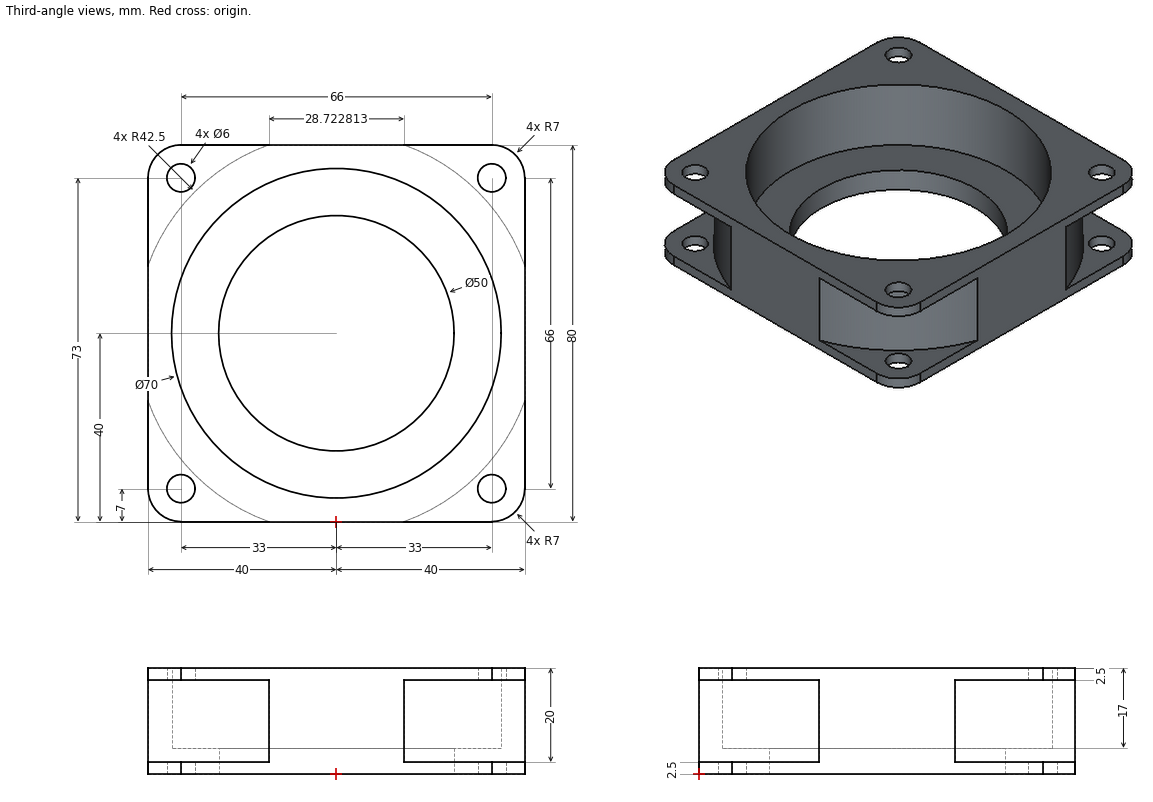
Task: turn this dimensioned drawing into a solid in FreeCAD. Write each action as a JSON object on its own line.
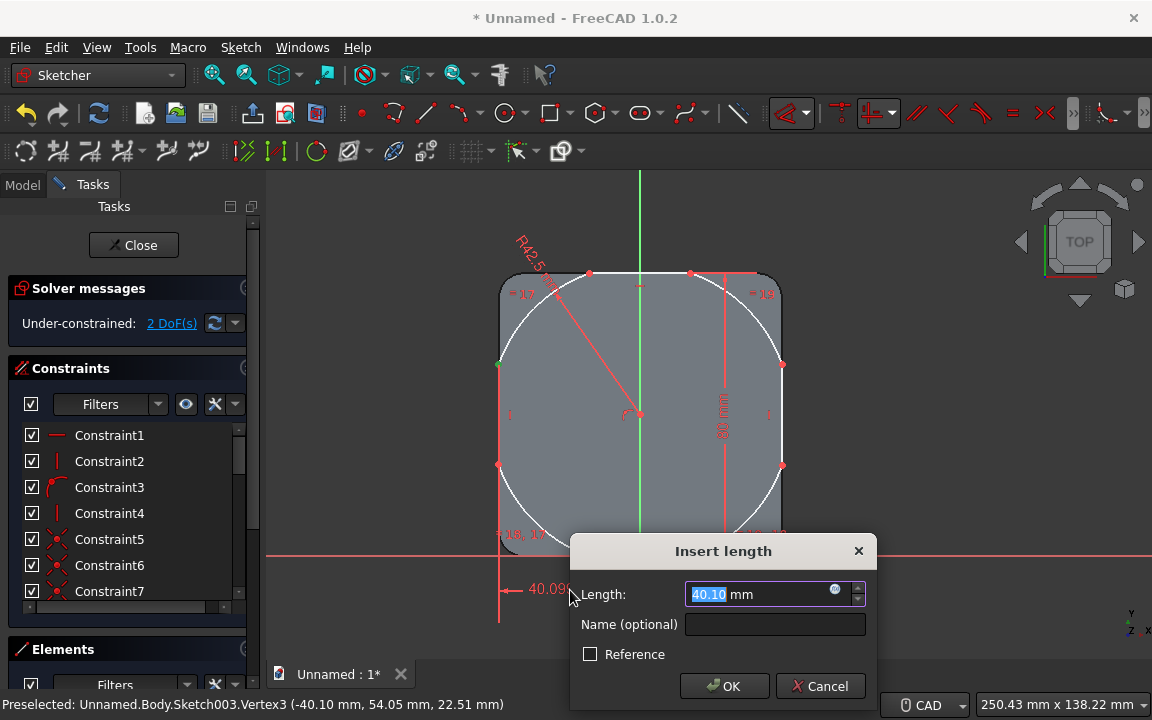
{"action": "type", "text": "40"}
{"action": "key", "text": "Return"}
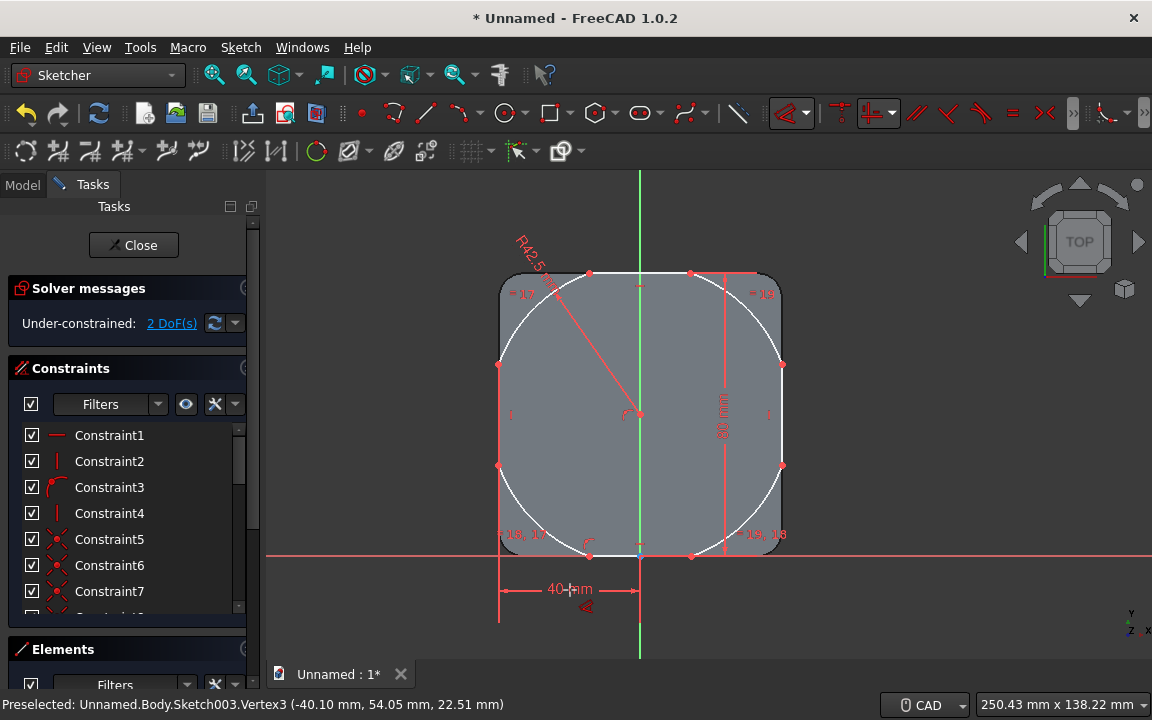
{"action": "left_click", "coordinate": [782, 465]}
{"action": "left_click", "coordinate": [711, 590]}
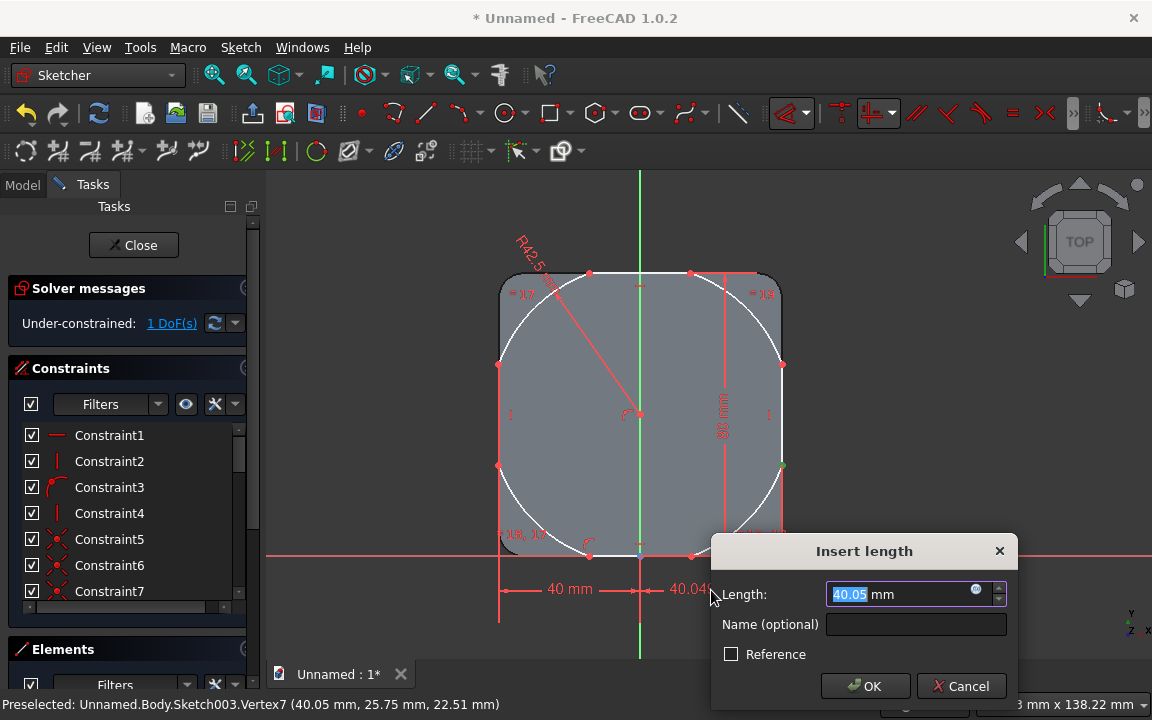
{"action": "type", "text": "40"}
{"action": "key", "text": "Return"}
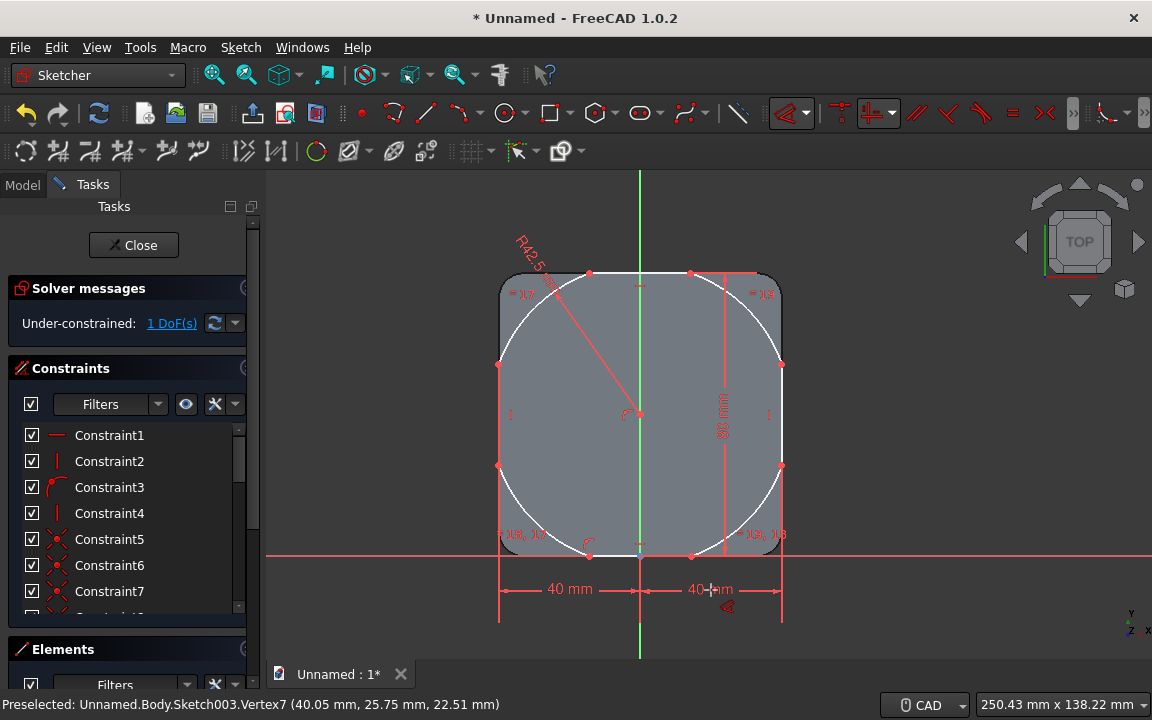
{"action": "left_click", "coordinate": [661, 273]}
{"action": "left_click", "coordinate": [617, 239]}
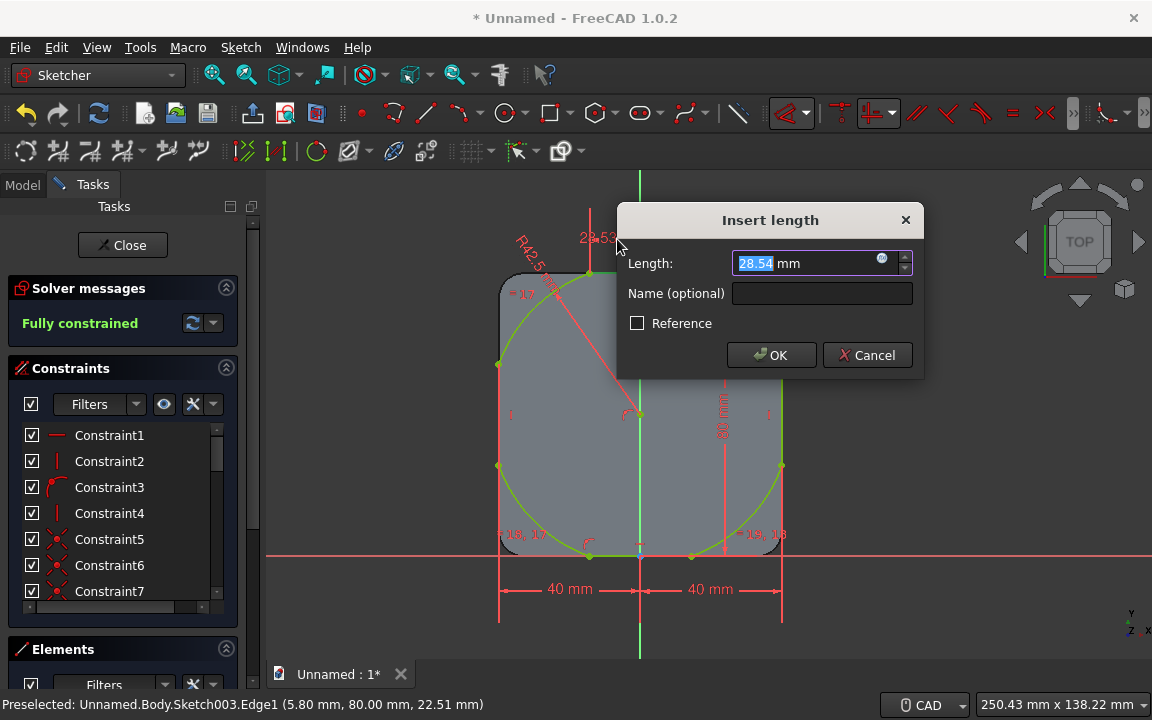
{"action": "type", "text": "28.722813"}
{"action": "key", "text": "Return"}
{"action": "key", "text": "Escape"}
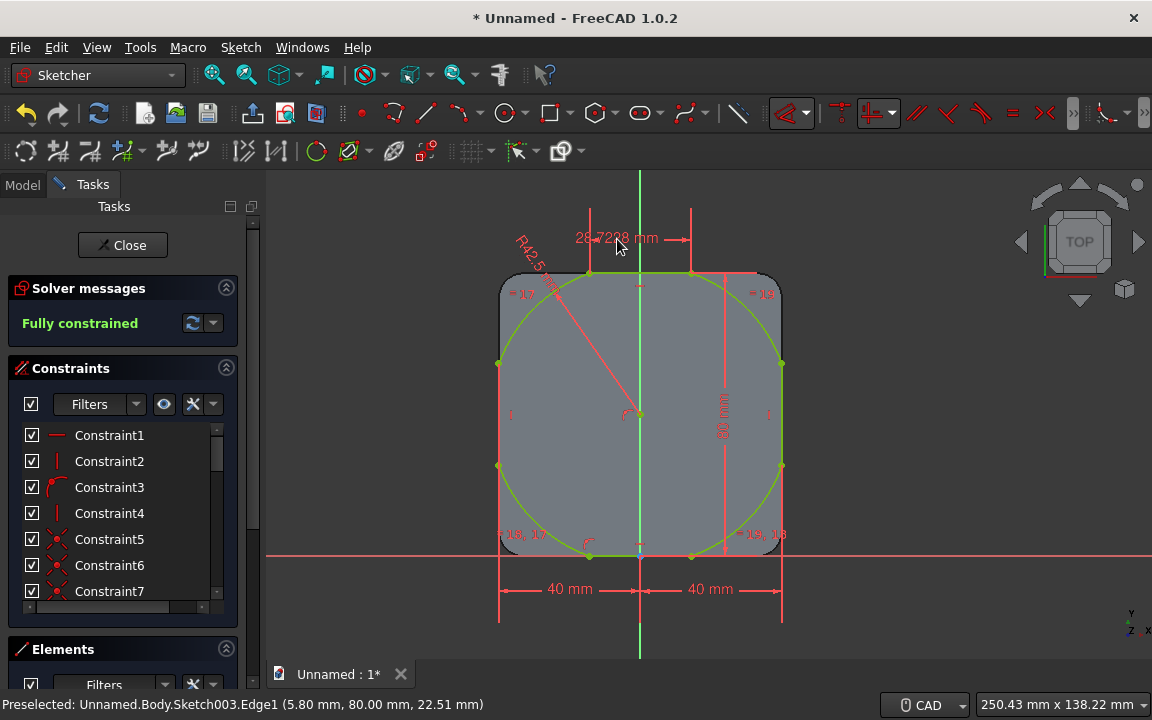
{"action": "left_click", "coordinate": [123, 245]}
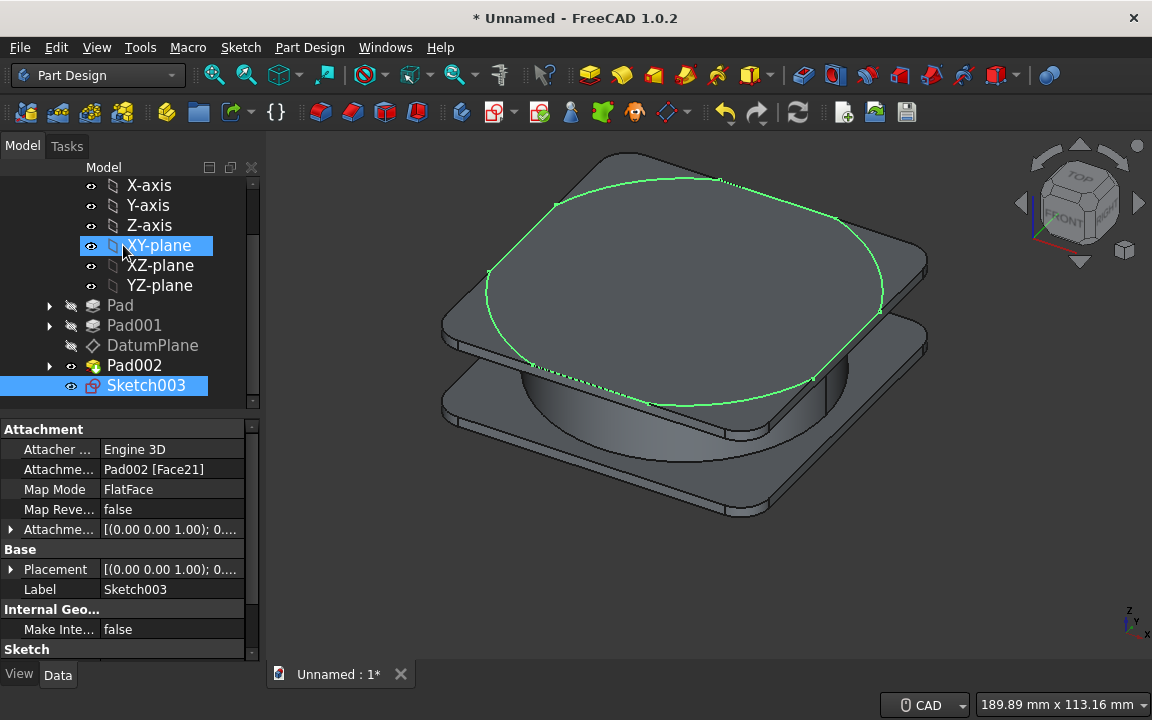
{"action": "left_click", "coordinate": [590, 76]}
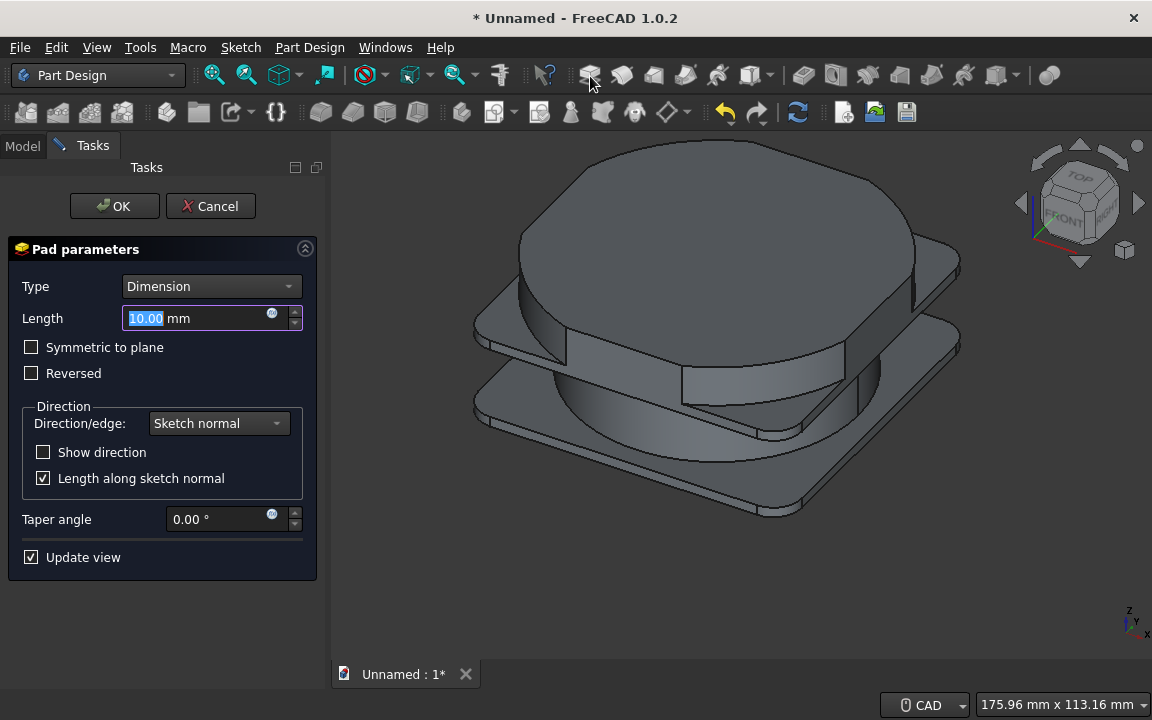
{"action": "type", "text": "20"}
{"action": "key", "text": "Tab"}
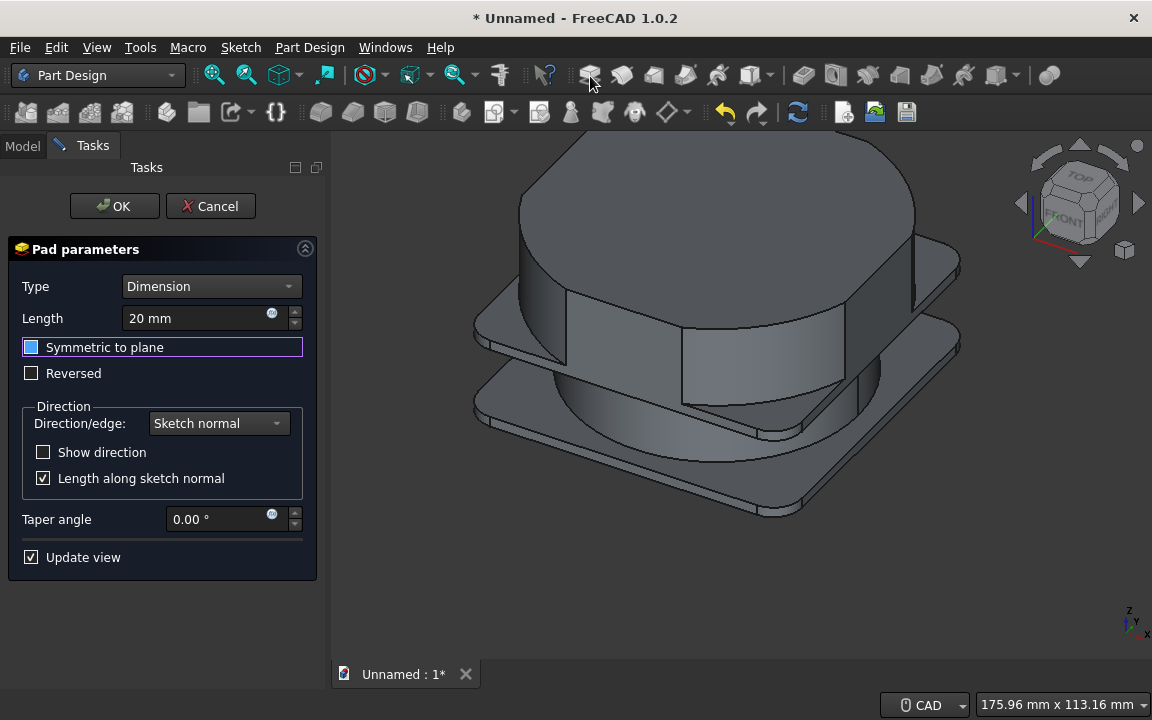
{"action": "left_click", "coordinate": [30, 373]}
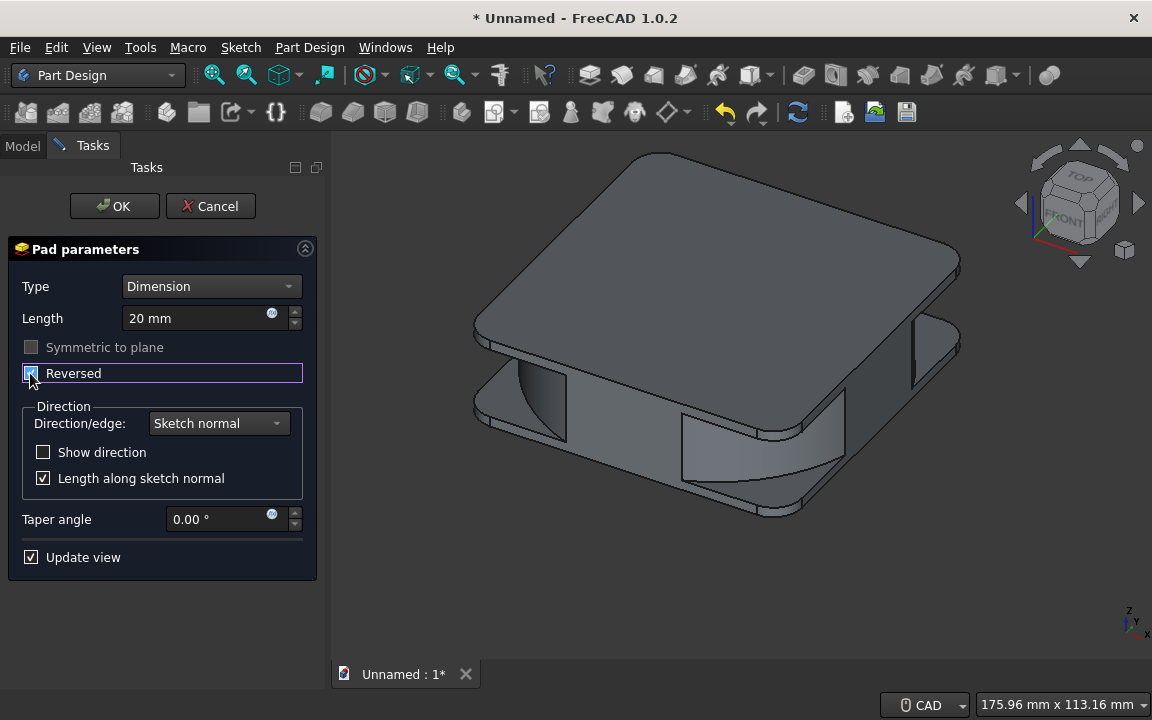
{"action": "left_click", "coordinate": [115, 206]}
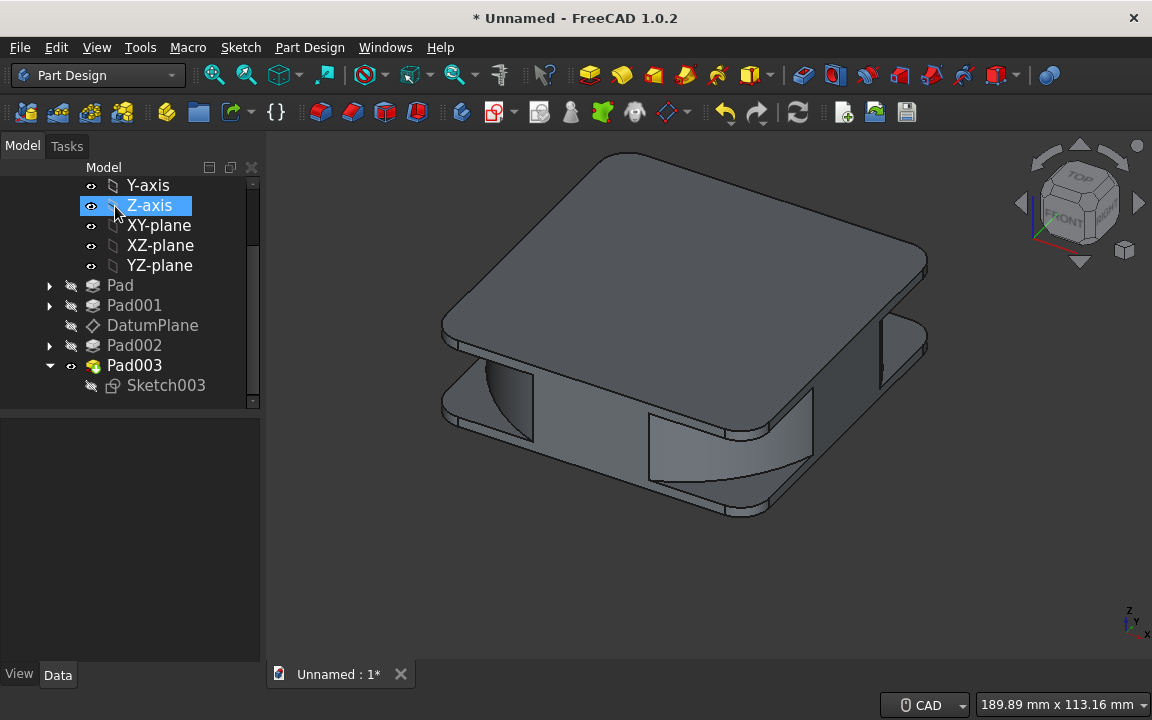
{"action": "left_click", "coordinate": [685, 291]}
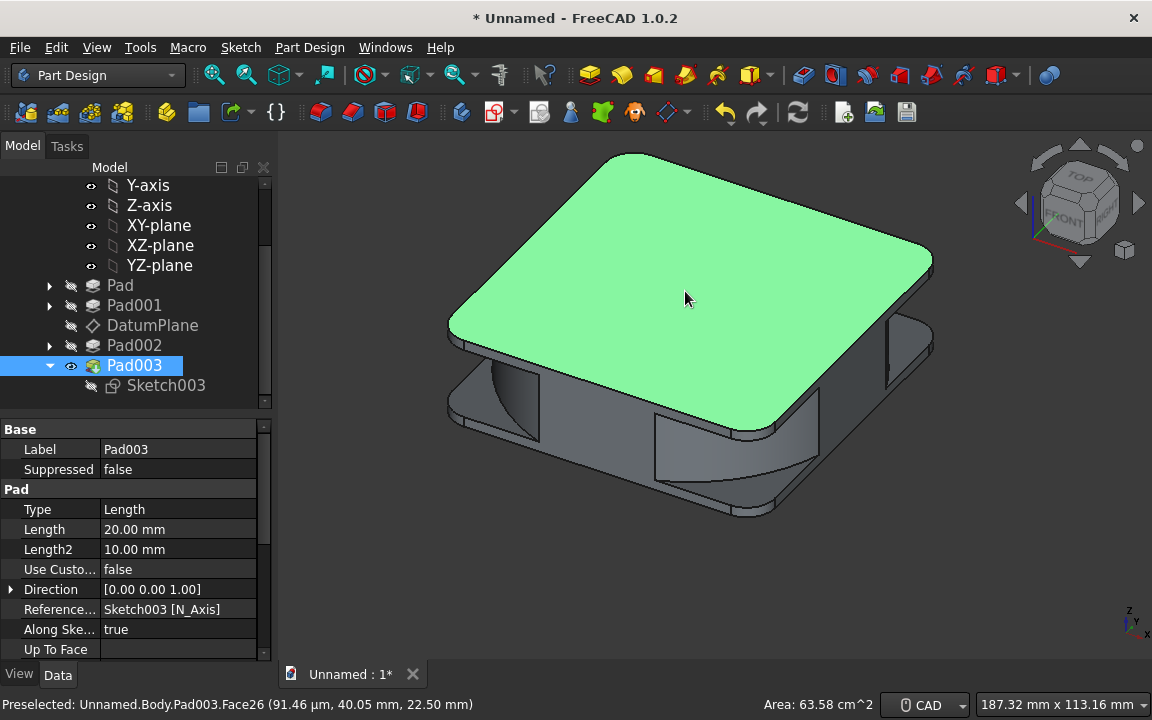
{"action": "left_click", "coordinate": [494, 112]}